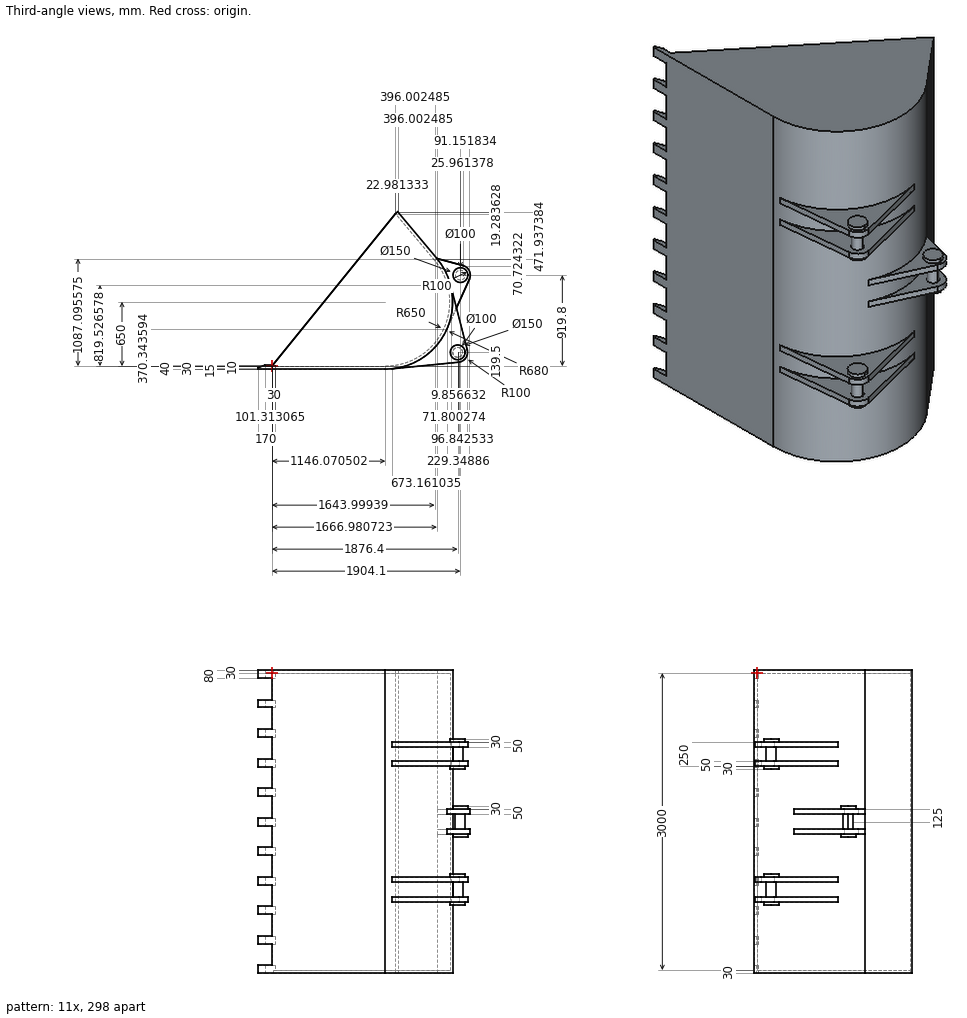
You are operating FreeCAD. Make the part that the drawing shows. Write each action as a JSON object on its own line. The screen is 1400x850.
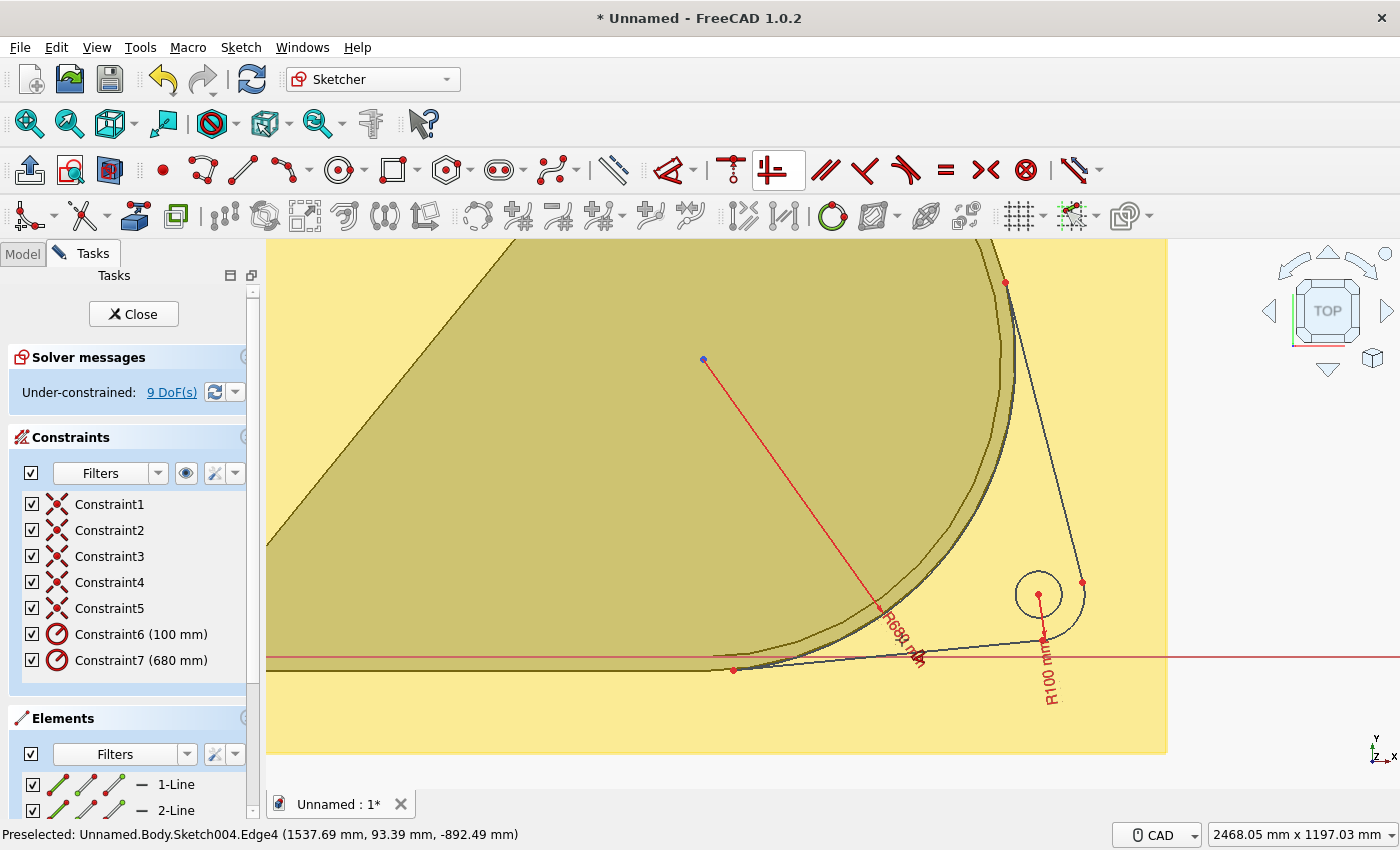
{"action": "left_click", "coordinate": [1055, 578]}
{"action": "left_click", "coordinate": [1054, 541]}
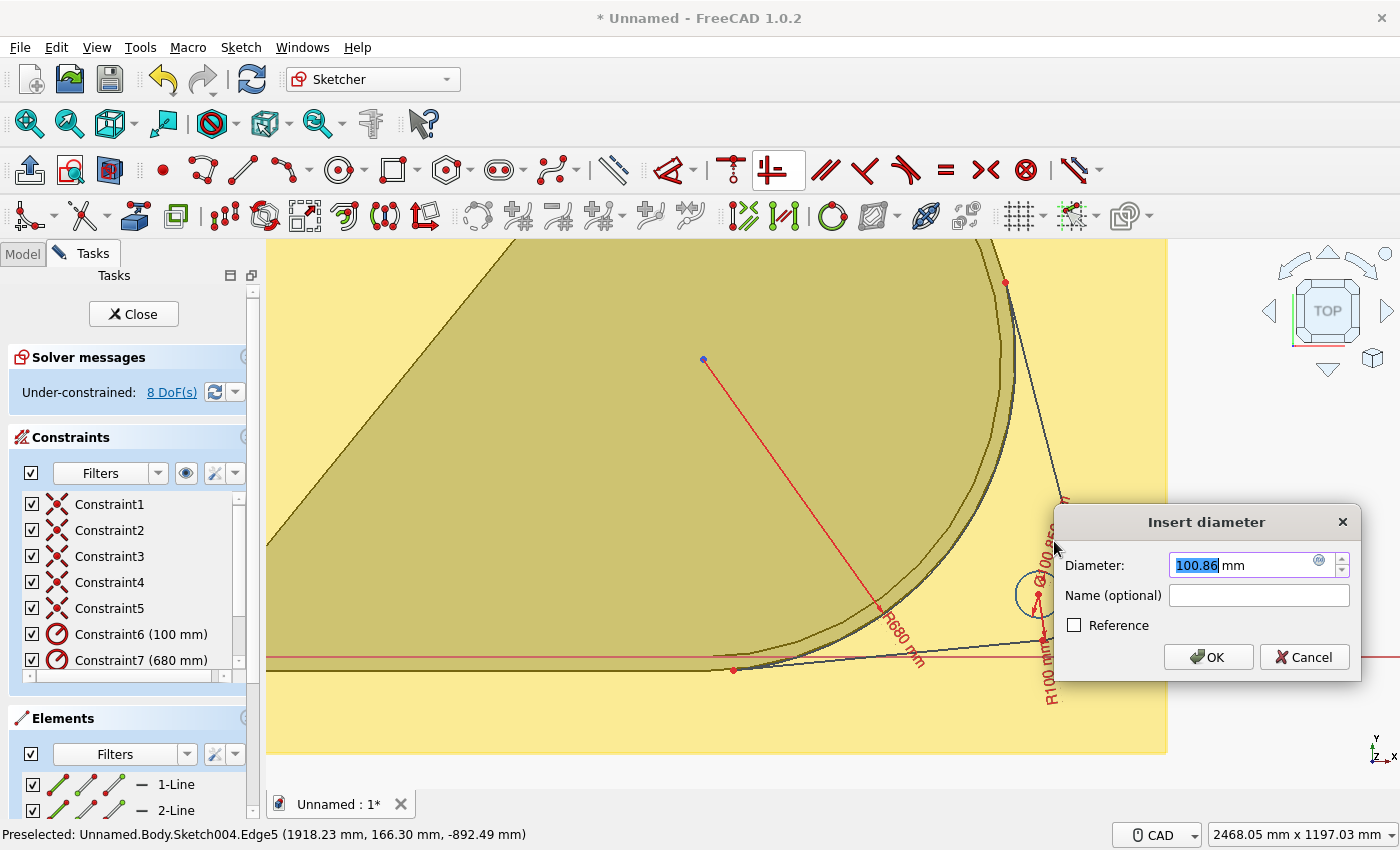
{"action": "type", "text": "100"}
{"action": "key", "text": "Return"}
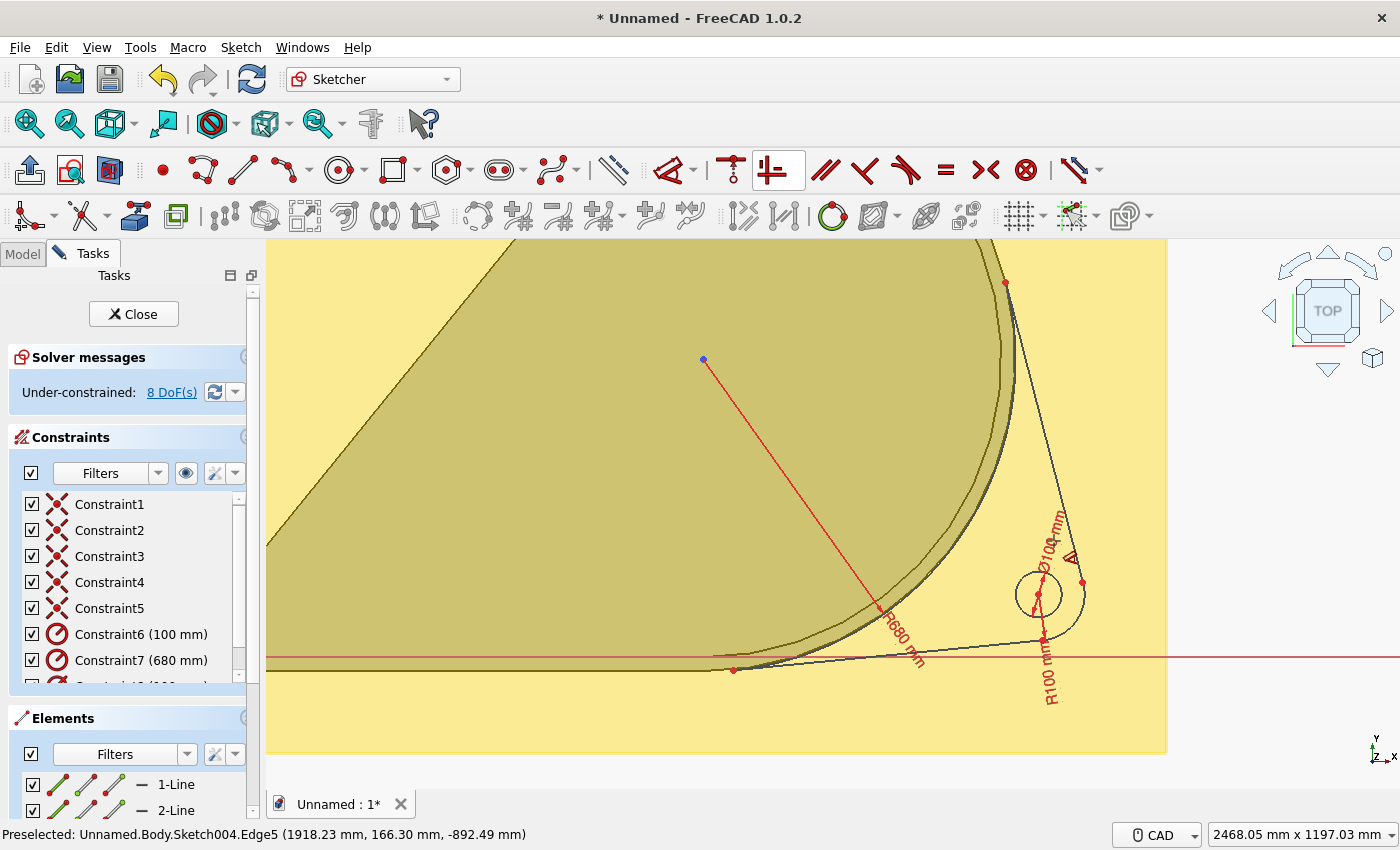
{"action": "left_click", "coordinate": [703, 359]}
{"action": "left_click", "coordinate": [737, 508]}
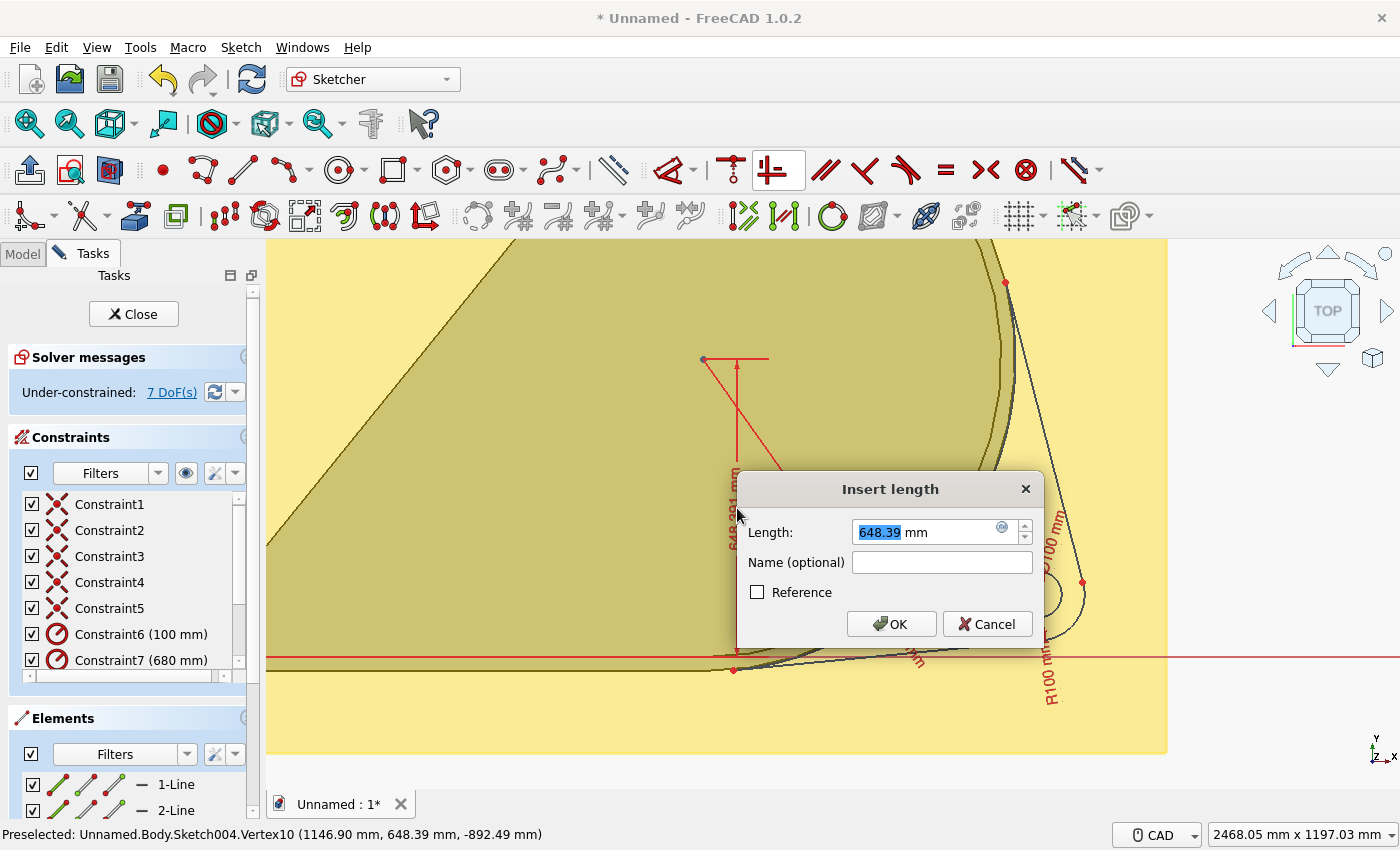
{"action": "type", "text": "650"}
{"action": "key", "text": "Return"}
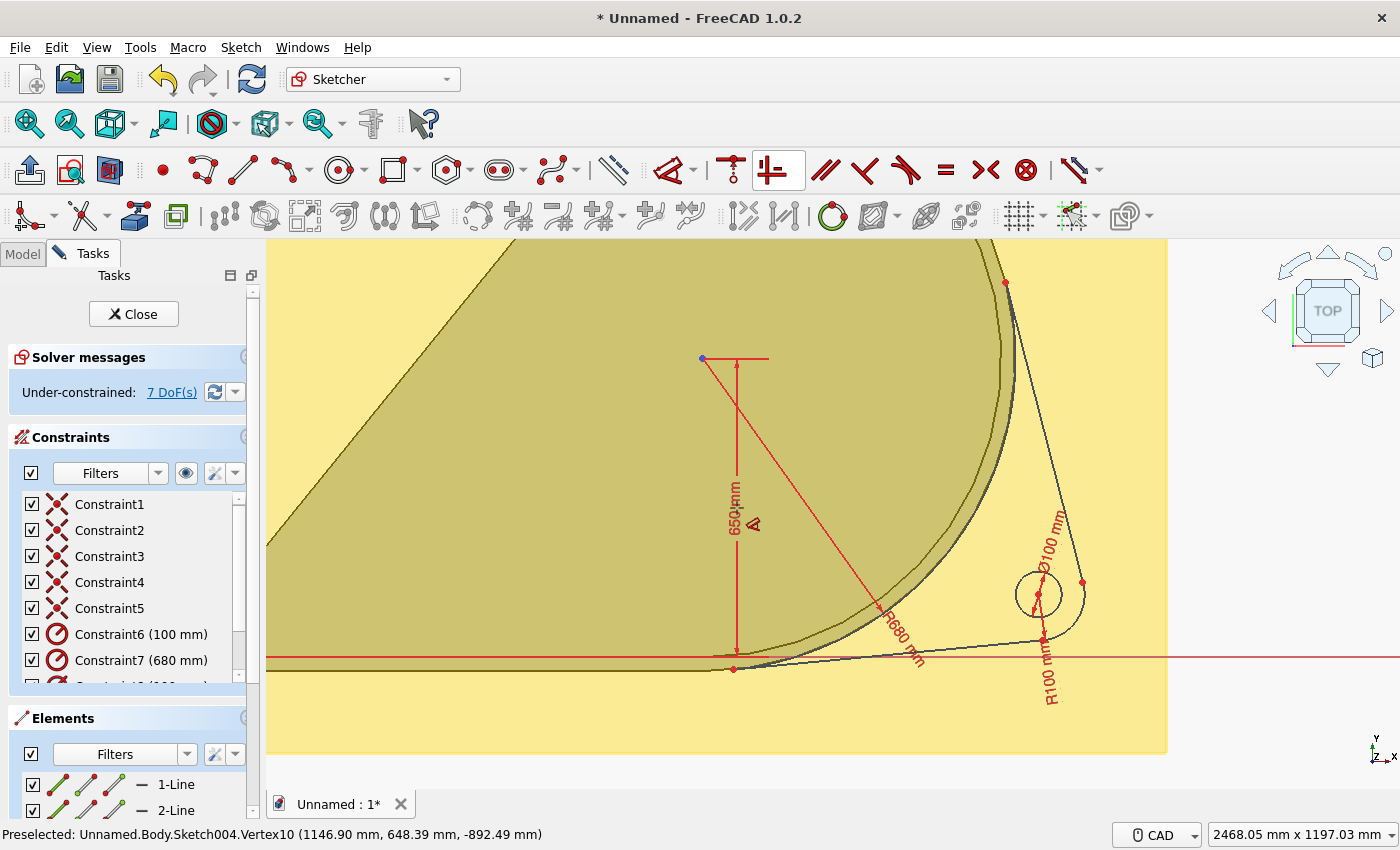
{"action": "left_click", "coordinate": [1039, 595]}
{"action": "left_click", "coordinate": [1097, 626]}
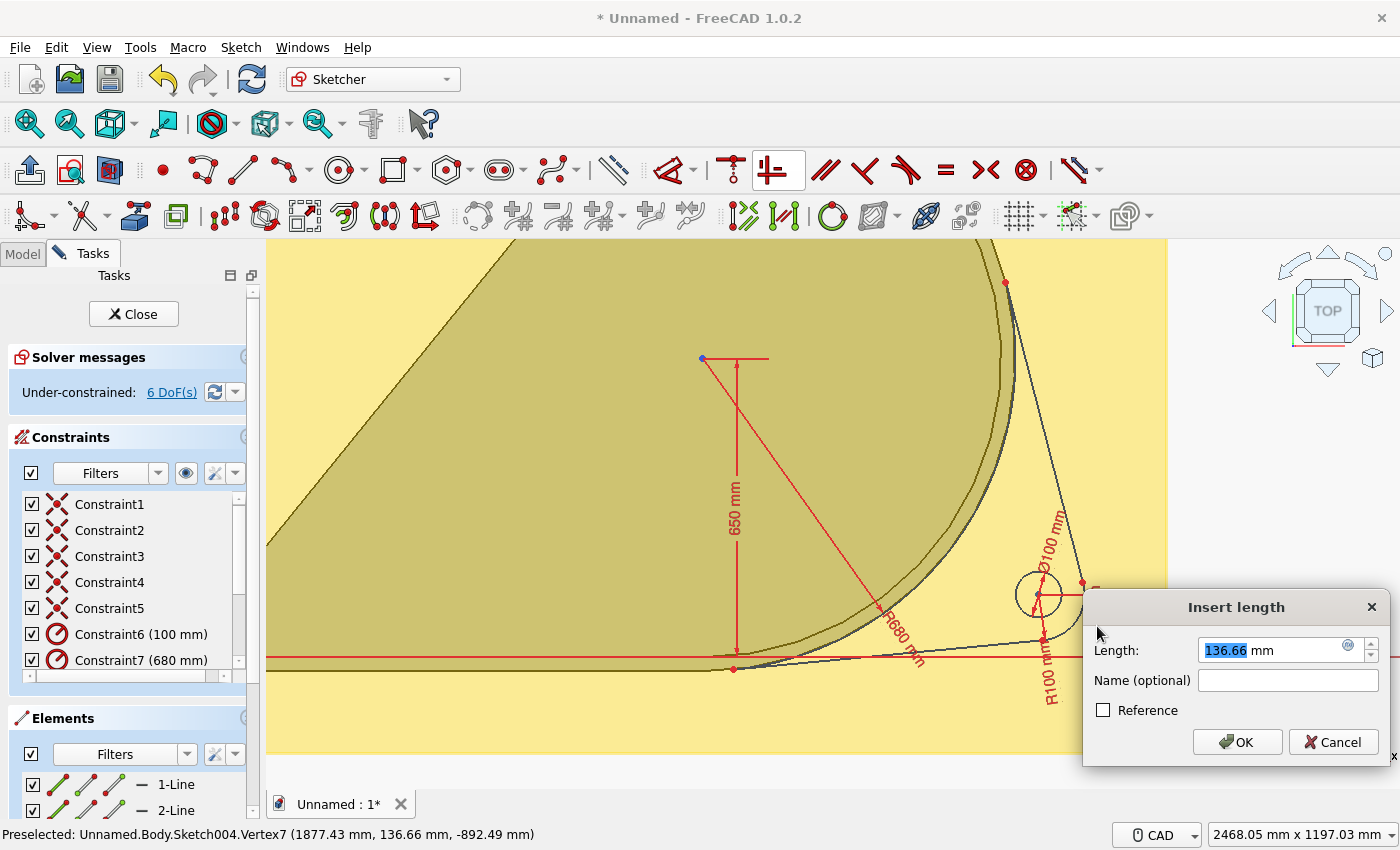
{"action": "type", "text": "139.5"}
{"action": "key", "text": "Return"}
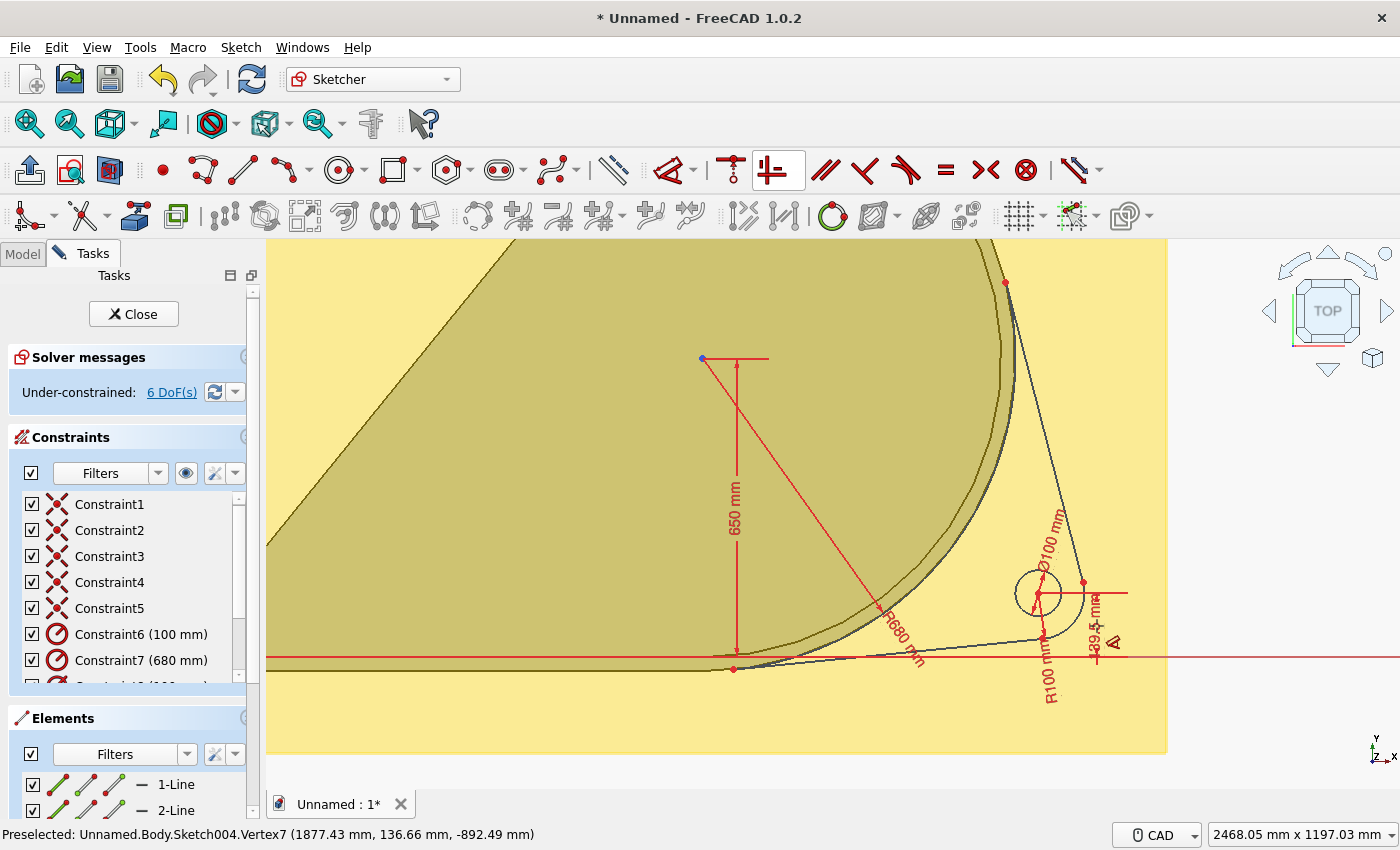
{"action": "left_click", "coordinate": [1038, 593]}
{"action": "left_click", "coordinate": [666, 691]}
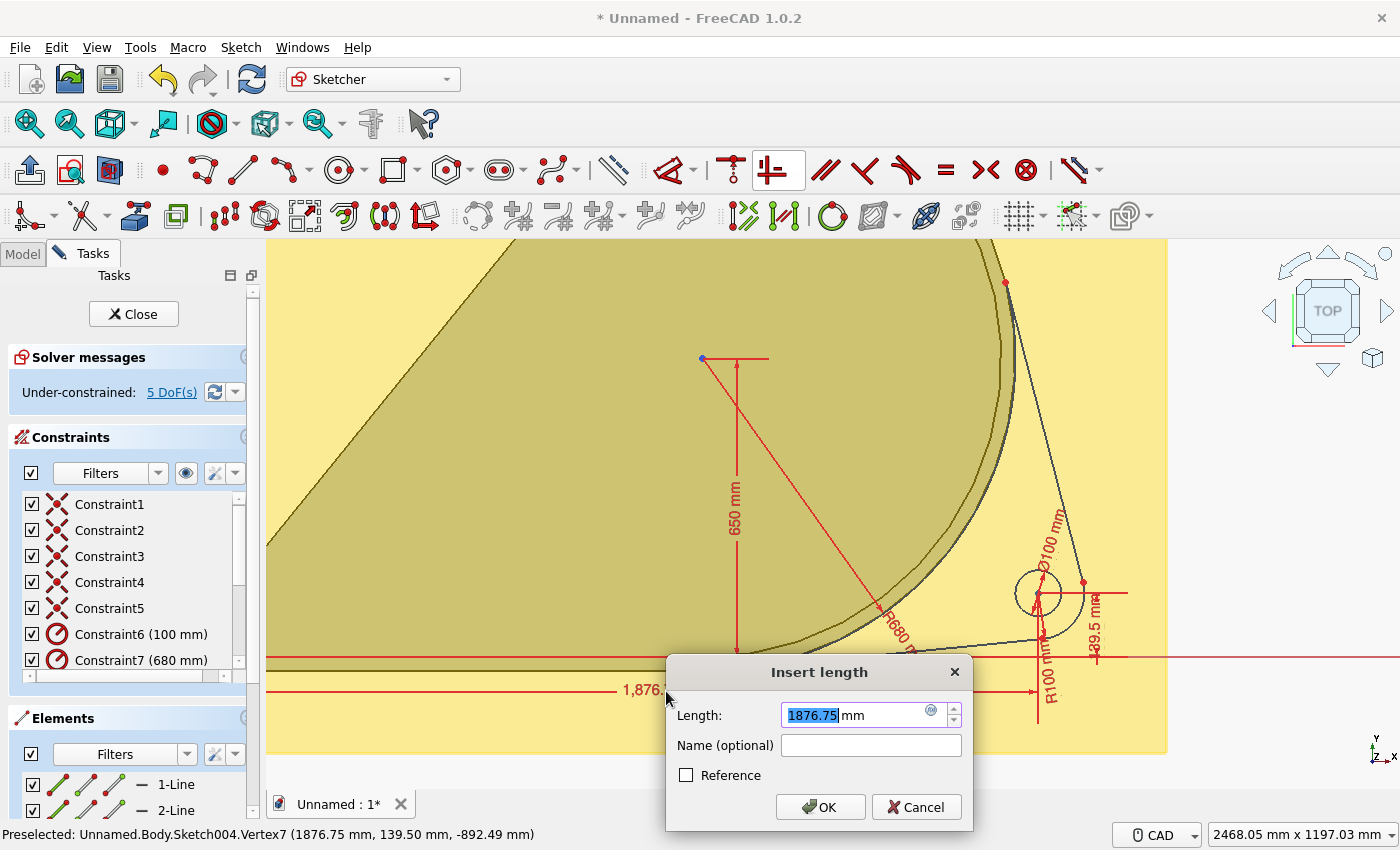
{"action": "type", "text": "1876.4"}
{"action": "key", "text": "Return"}